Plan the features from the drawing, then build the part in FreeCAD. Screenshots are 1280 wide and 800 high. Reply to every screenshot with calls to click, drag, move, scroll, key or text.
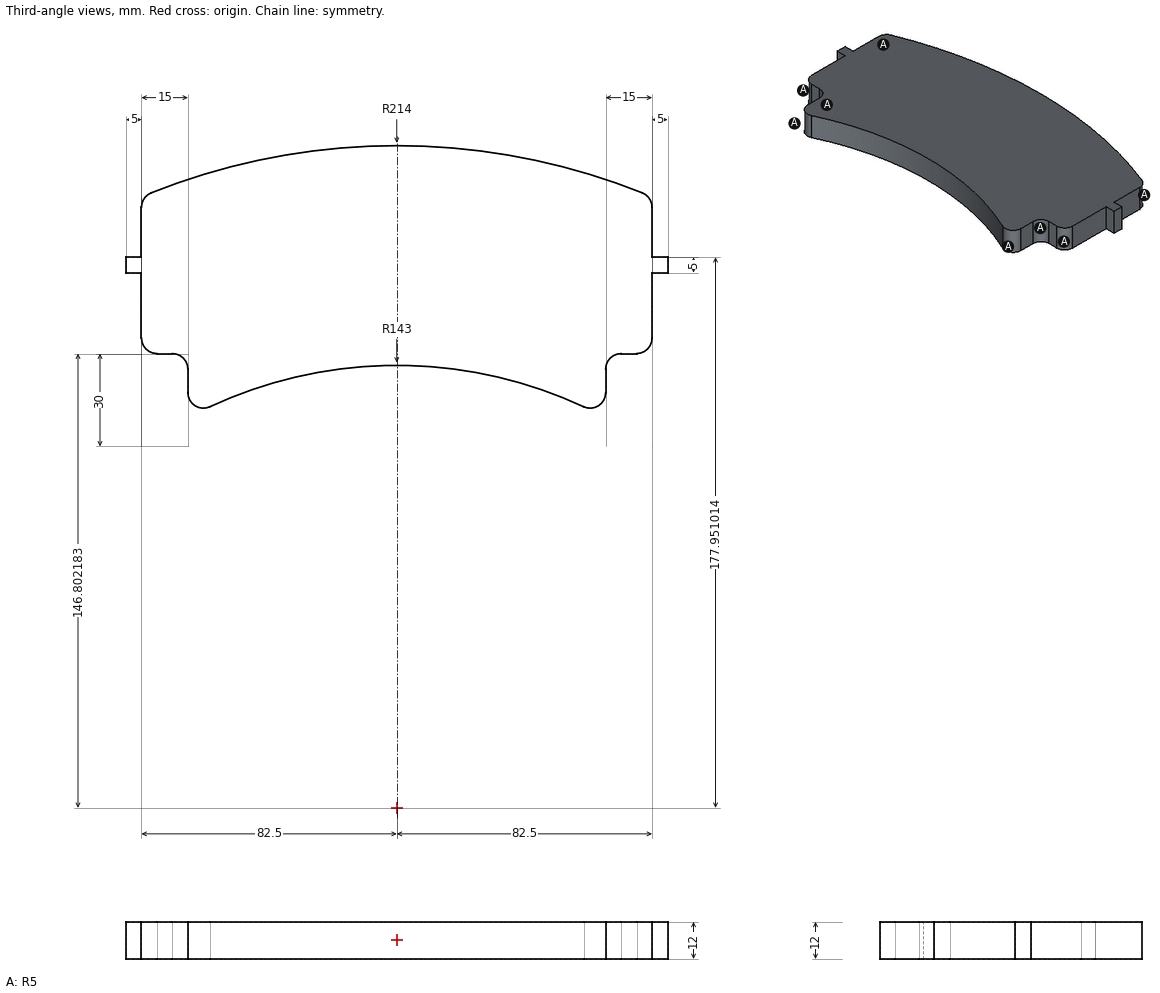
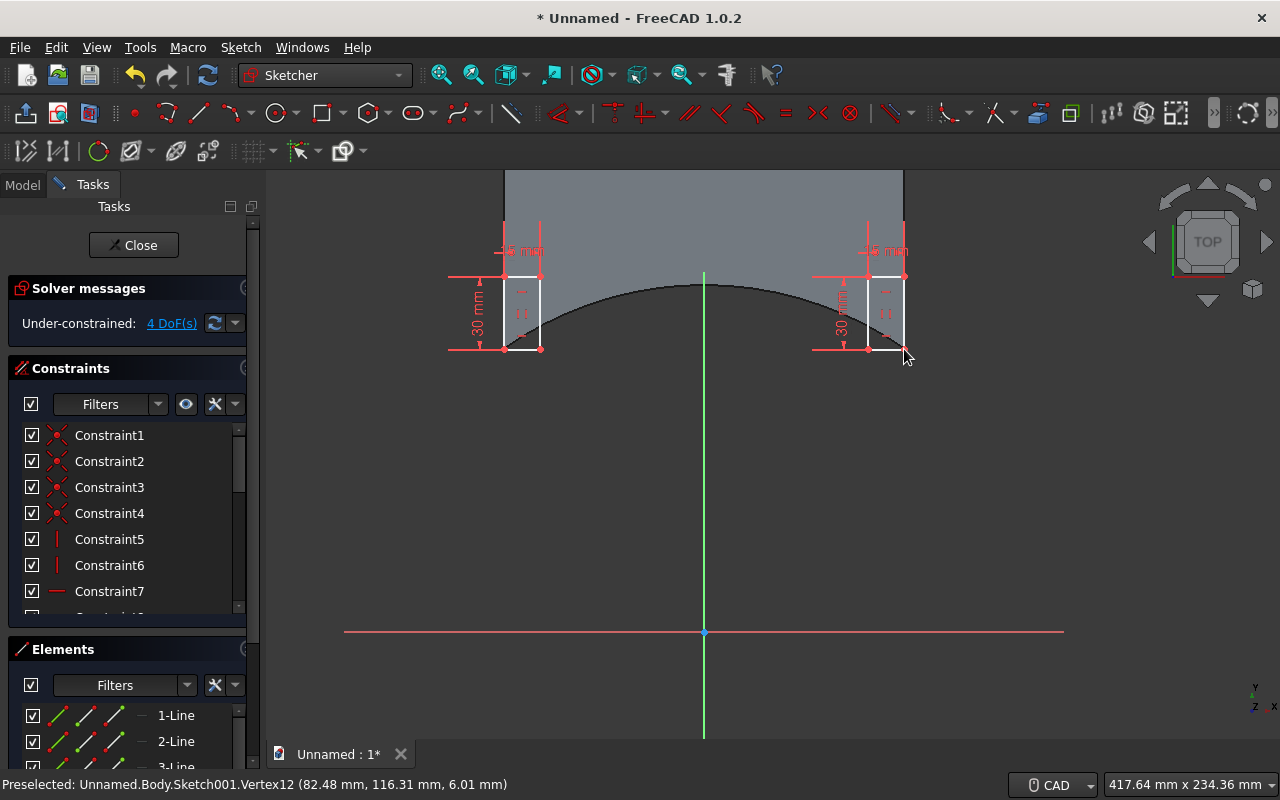
click(540, 277)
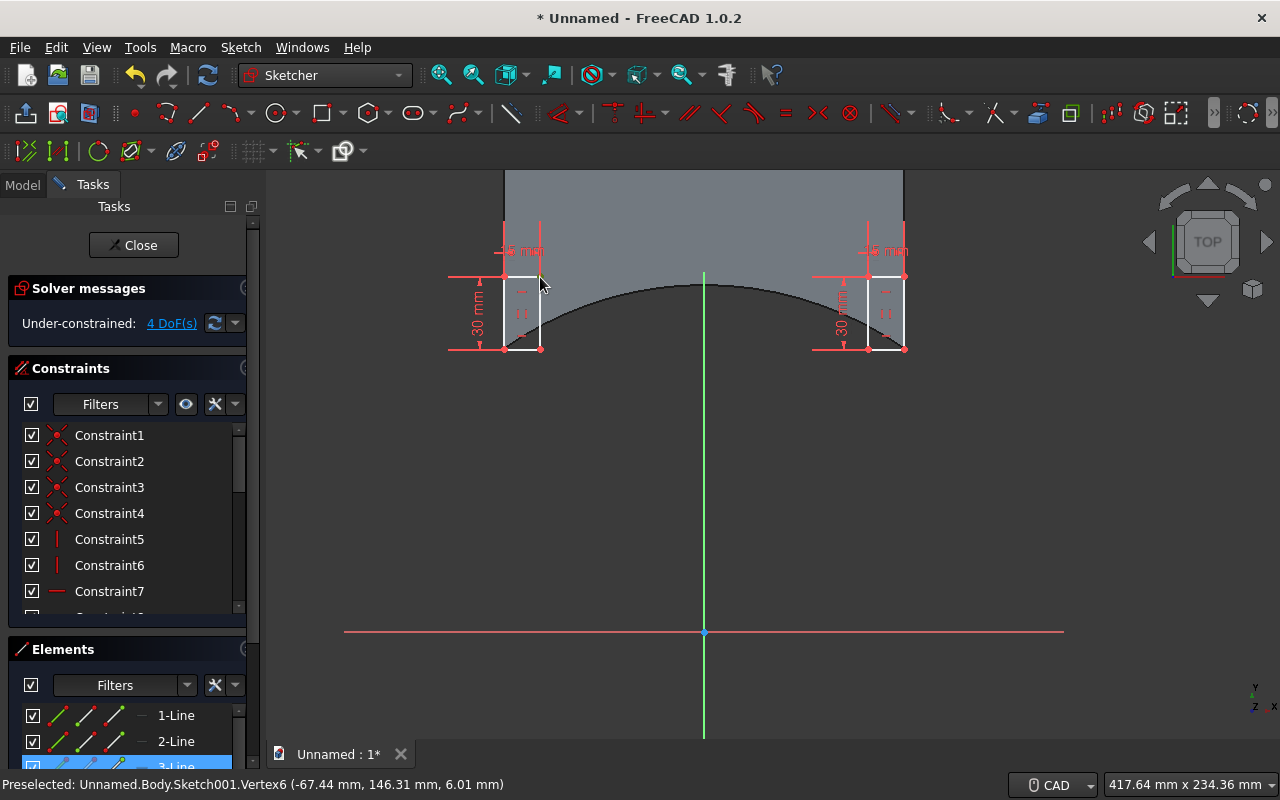
click(868, 277)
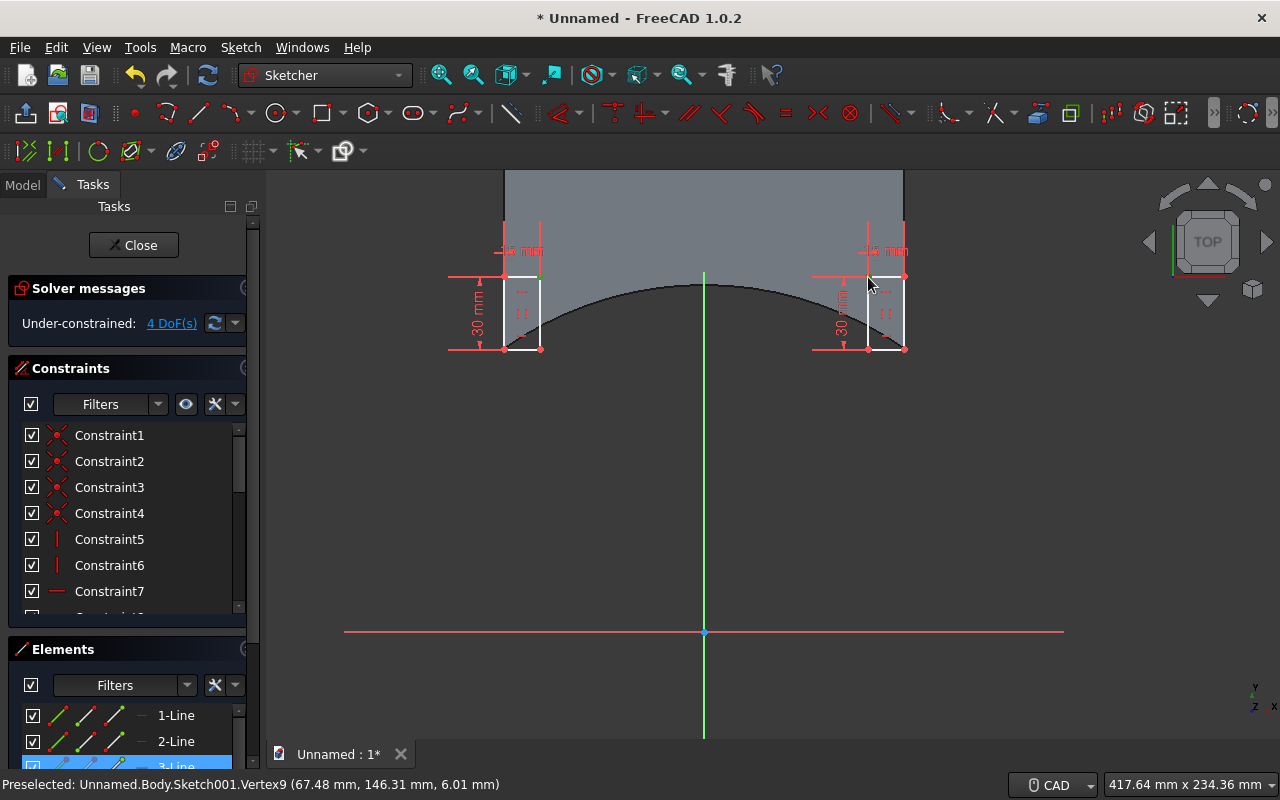
click(704, 674)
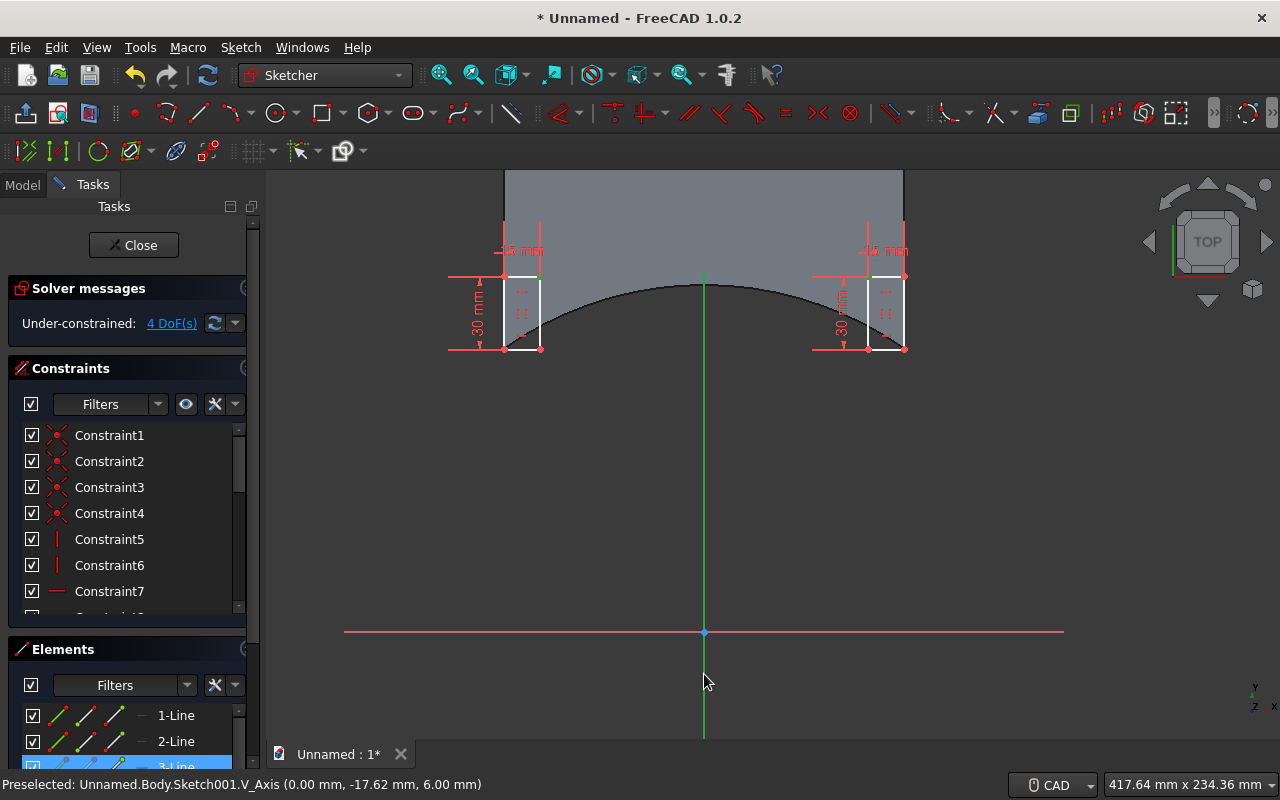
click(818, 114)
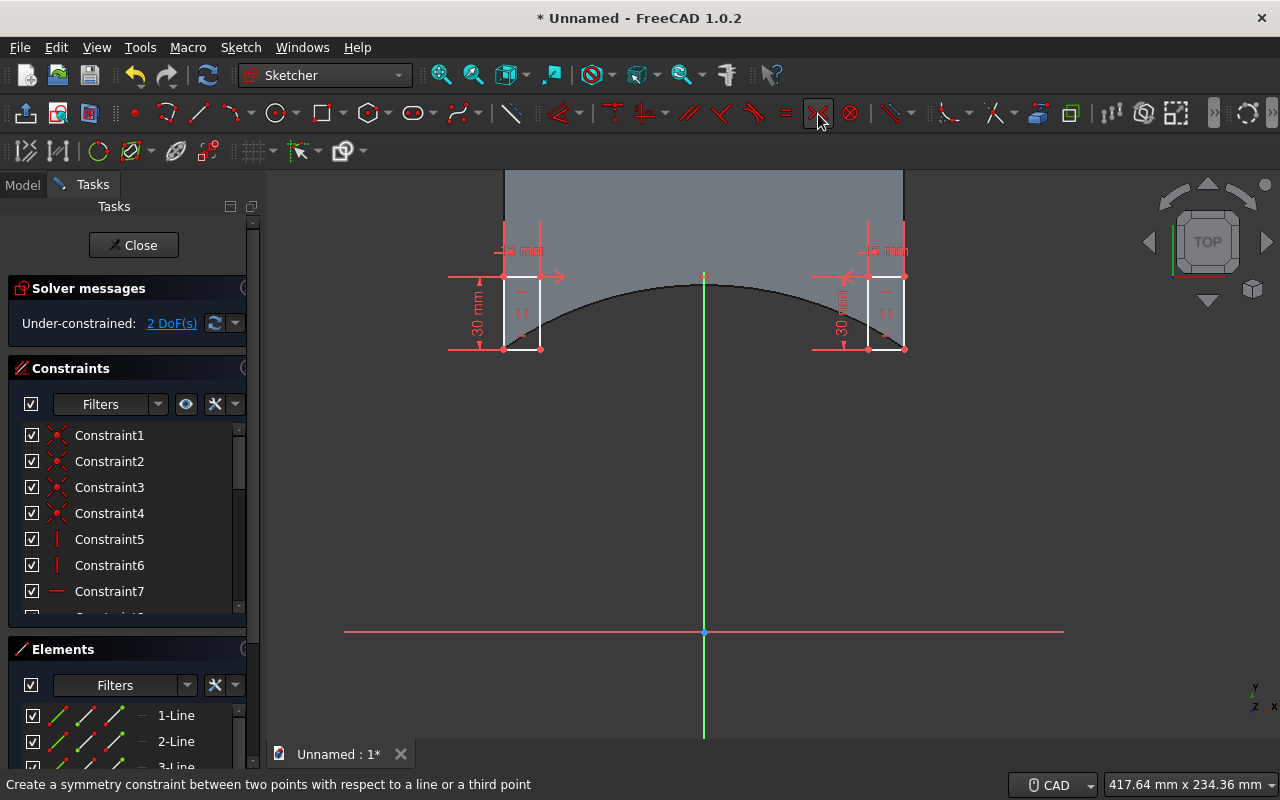
click(558, 114)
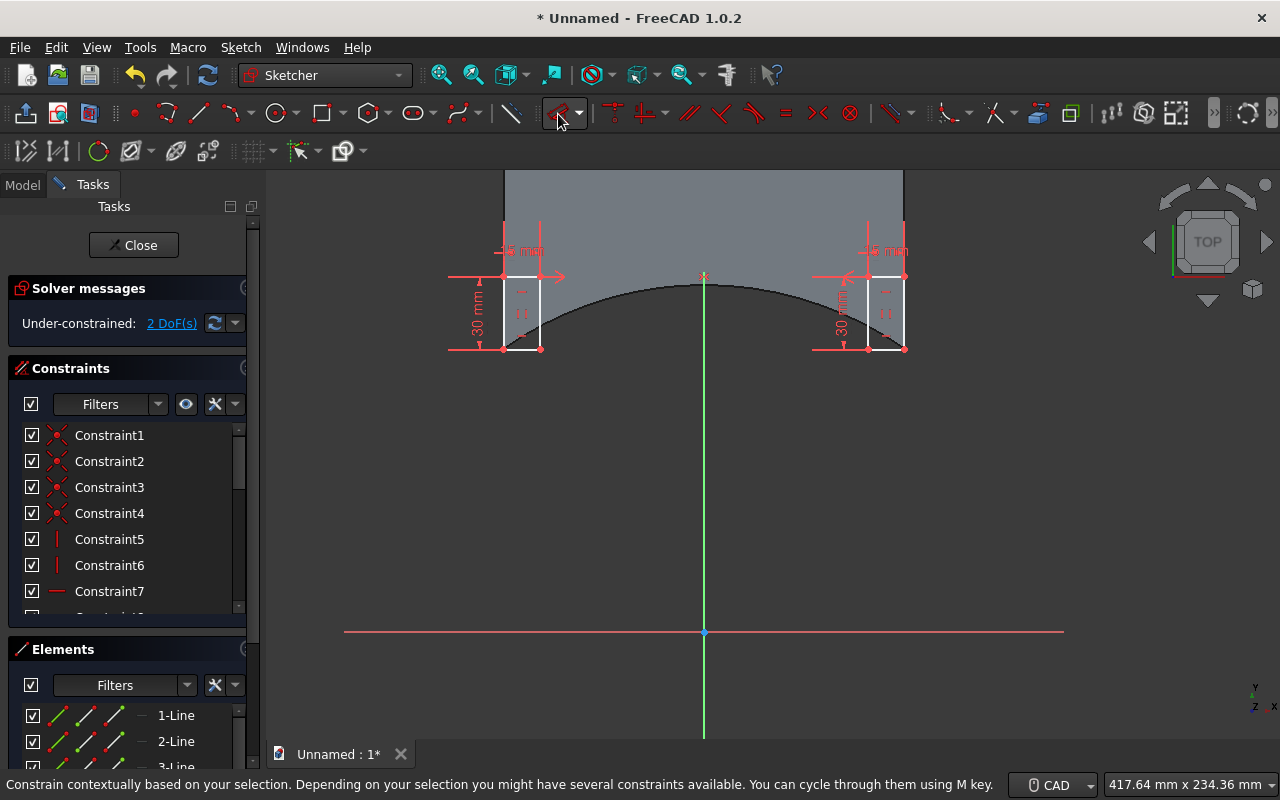
click(504, 277)
click(604, 666)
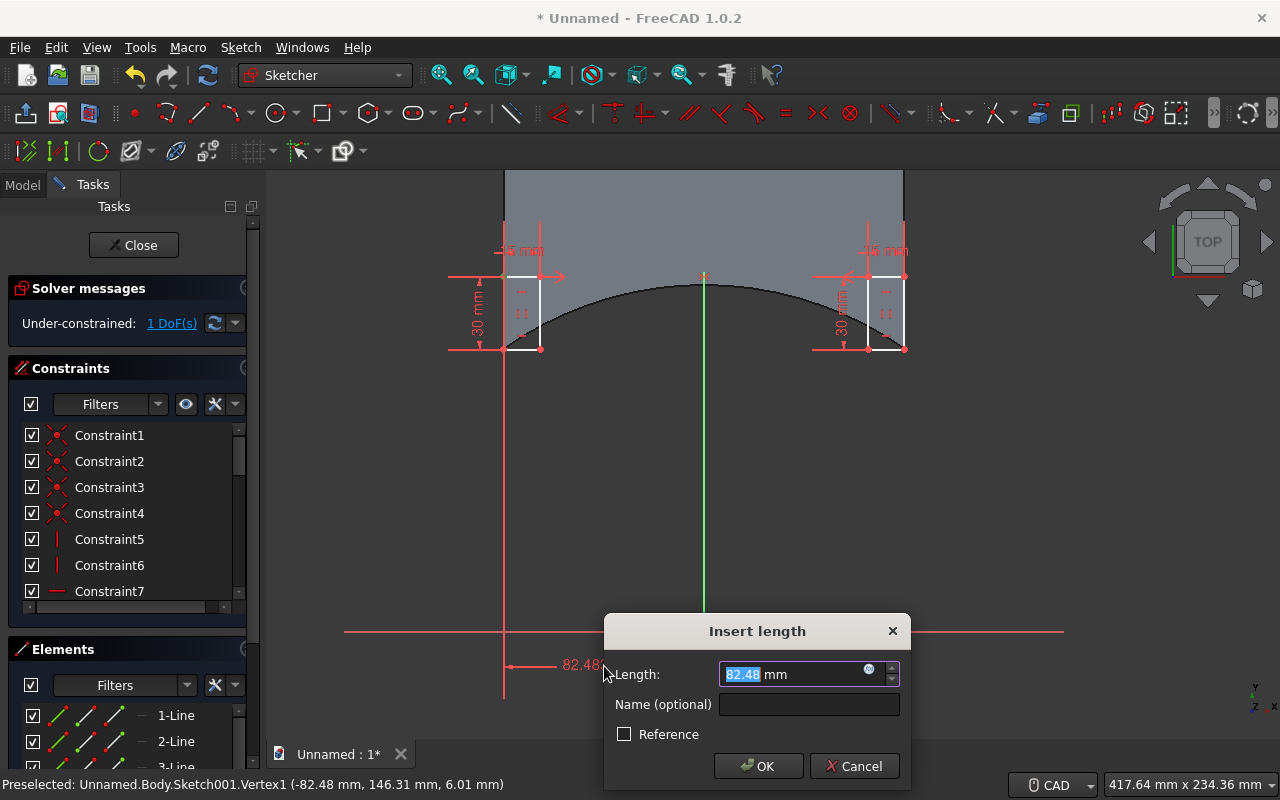
text(82.5)
key(Return)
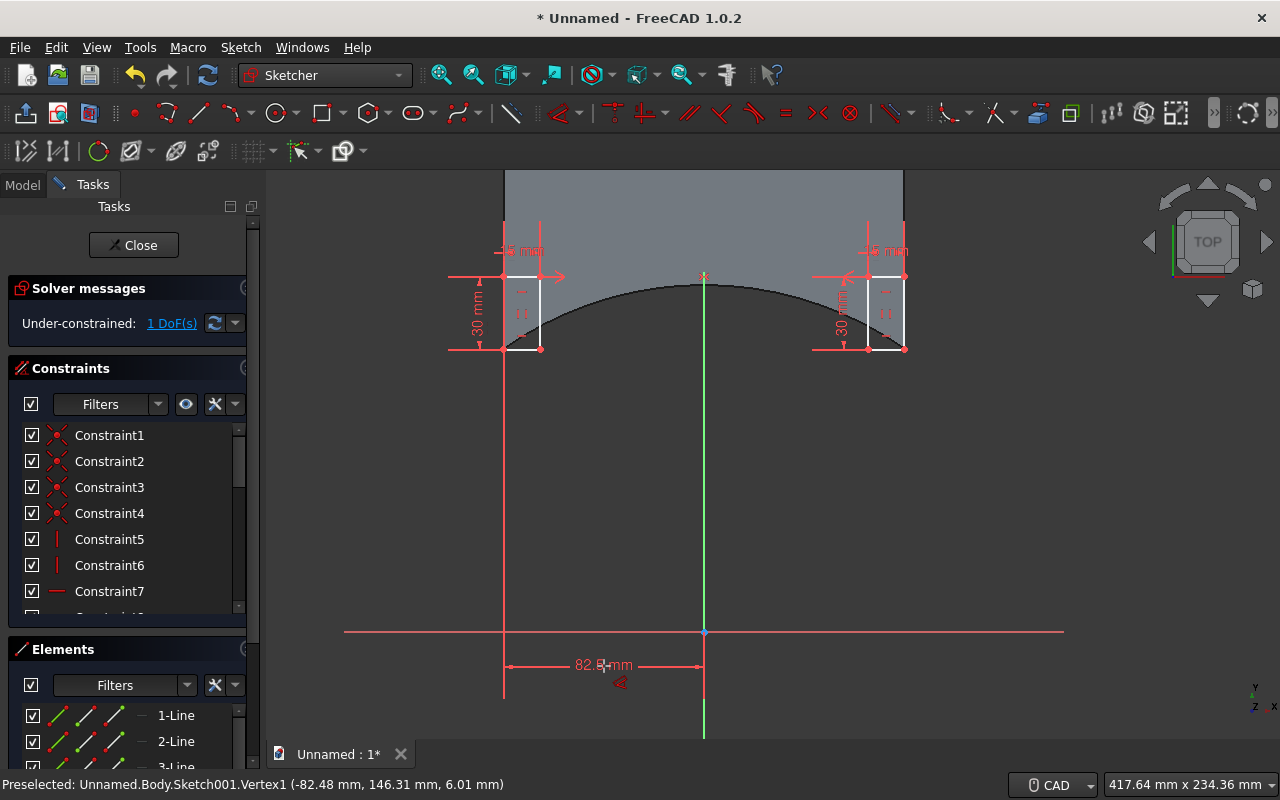
click(504, 277)
click(470, 455)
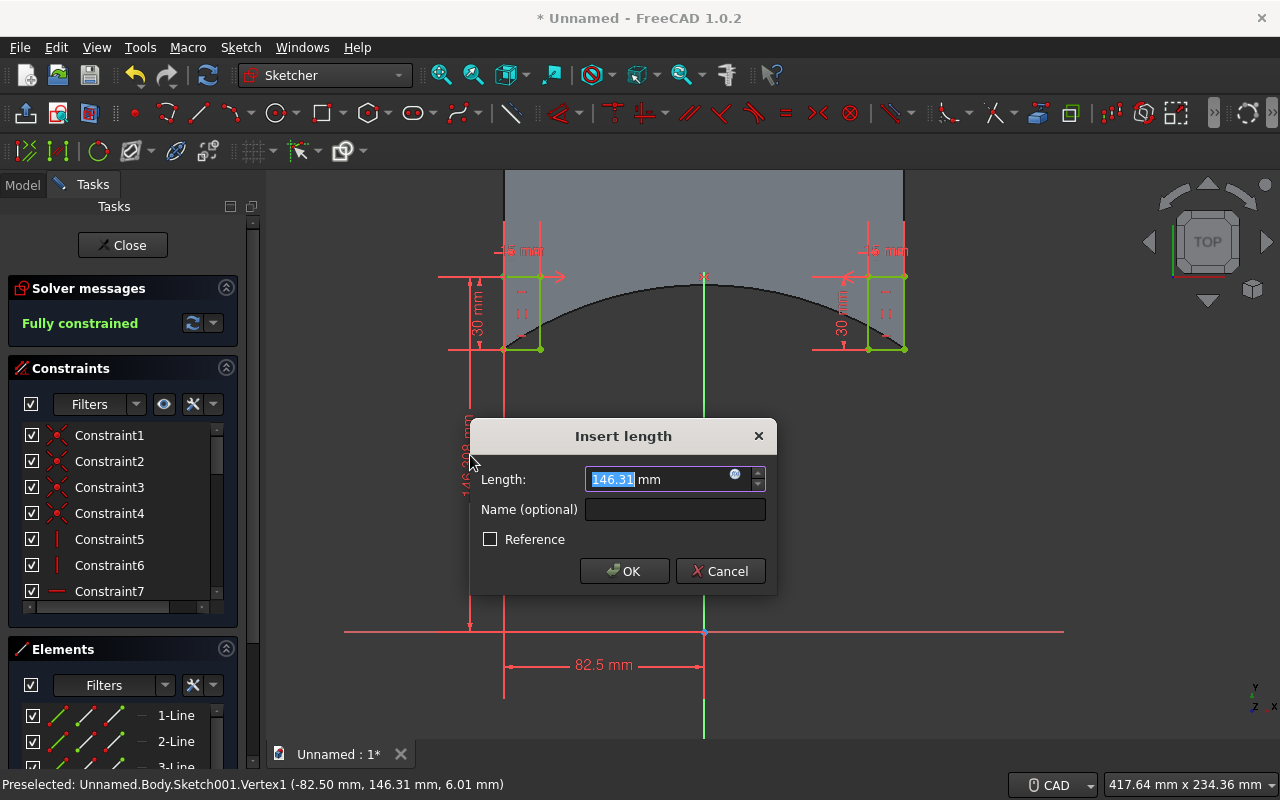
text(146.802183)
key(Return)
key(Escape)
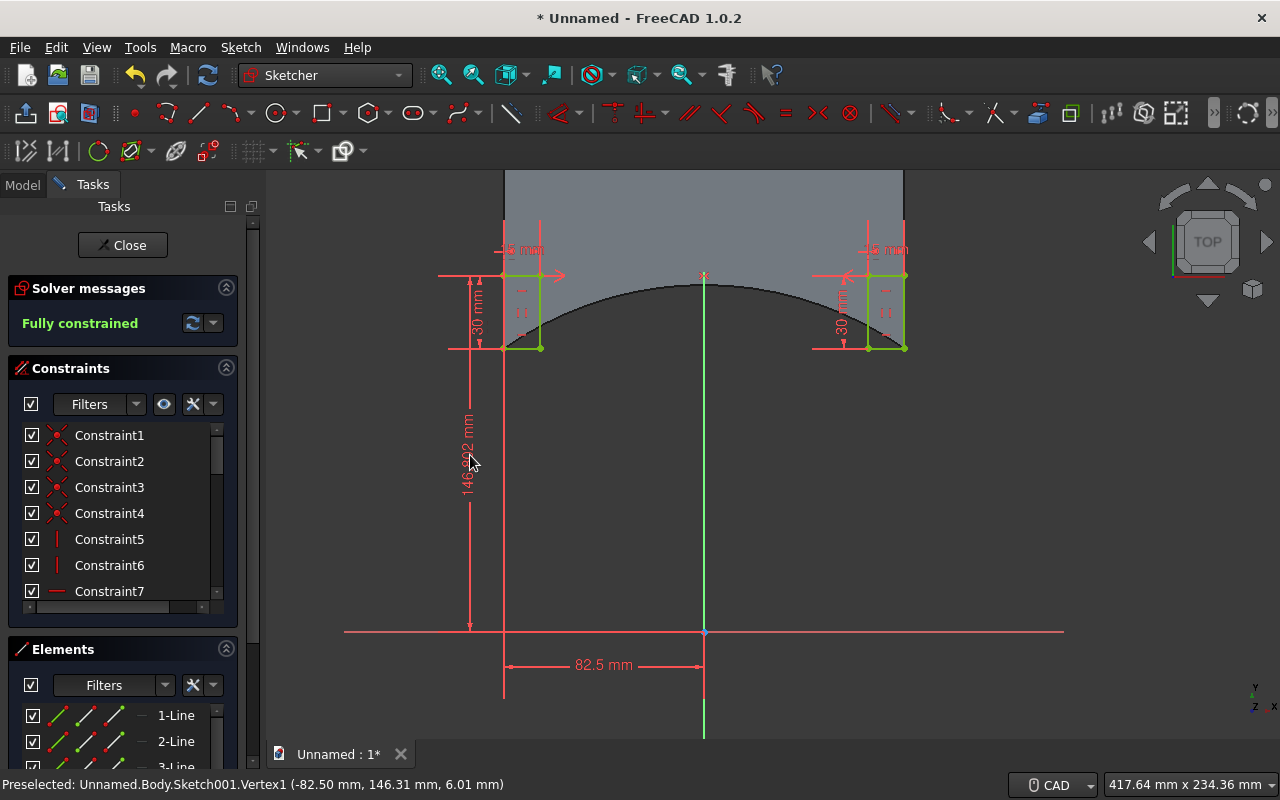
click(123, 245)